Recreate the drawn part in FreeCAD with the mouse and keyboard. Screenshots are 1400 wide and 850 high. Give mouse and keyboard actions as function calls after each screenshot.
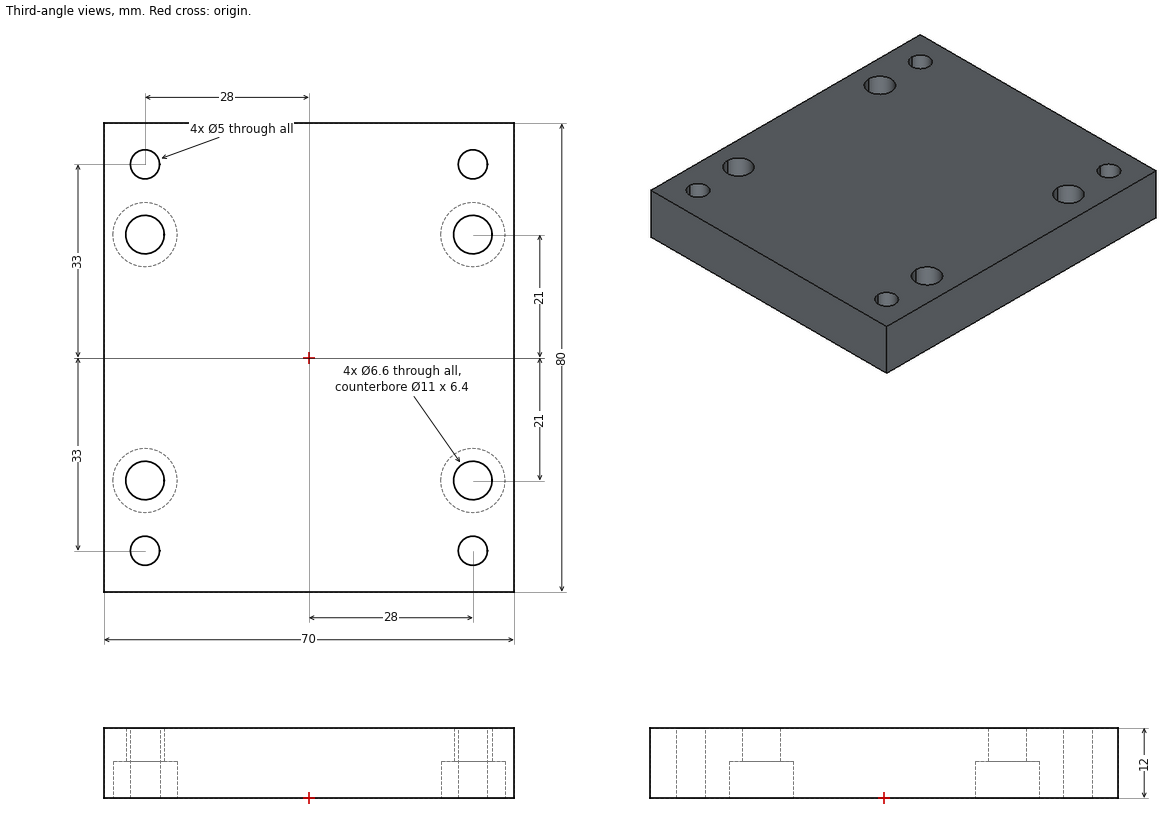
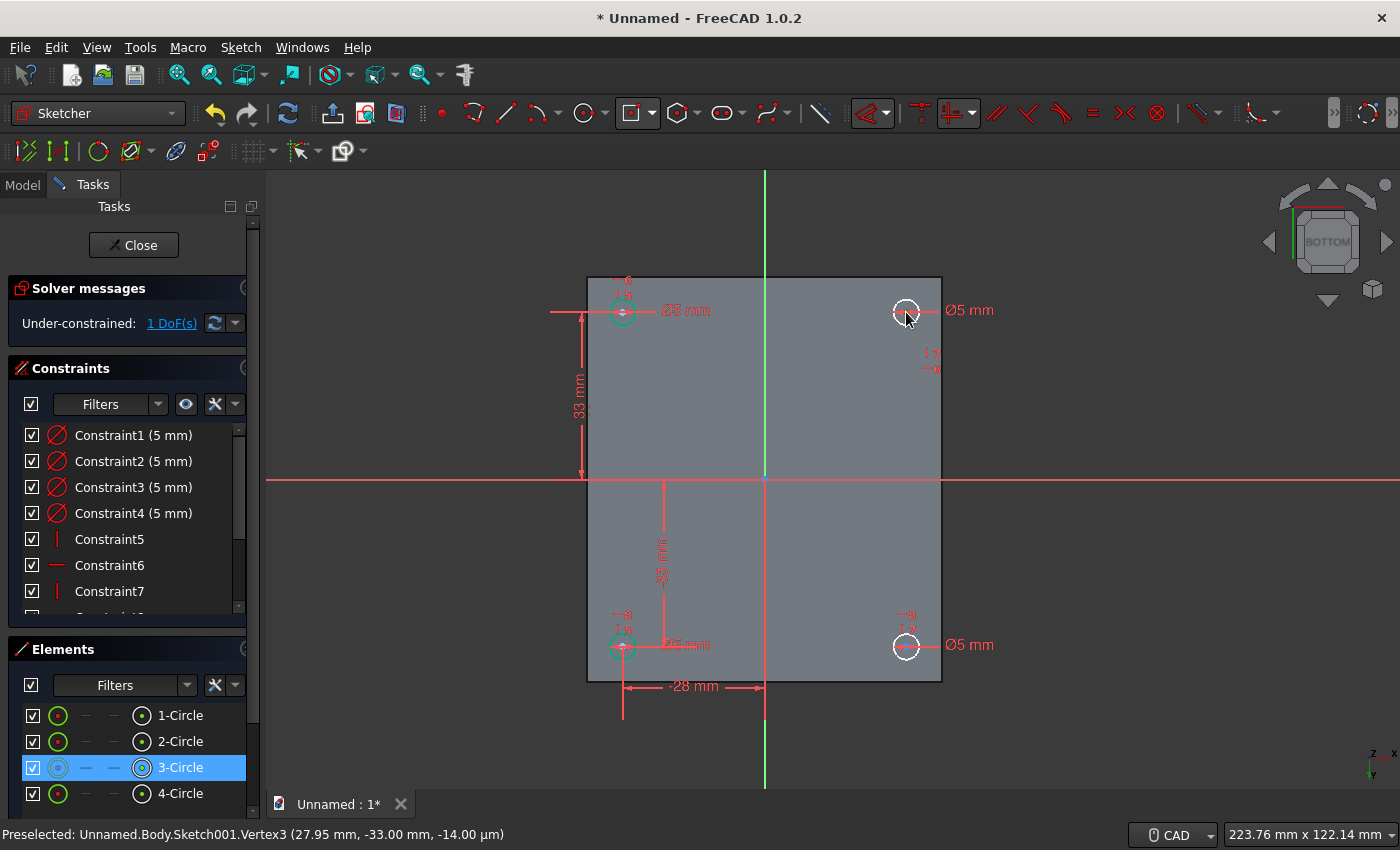
key(l)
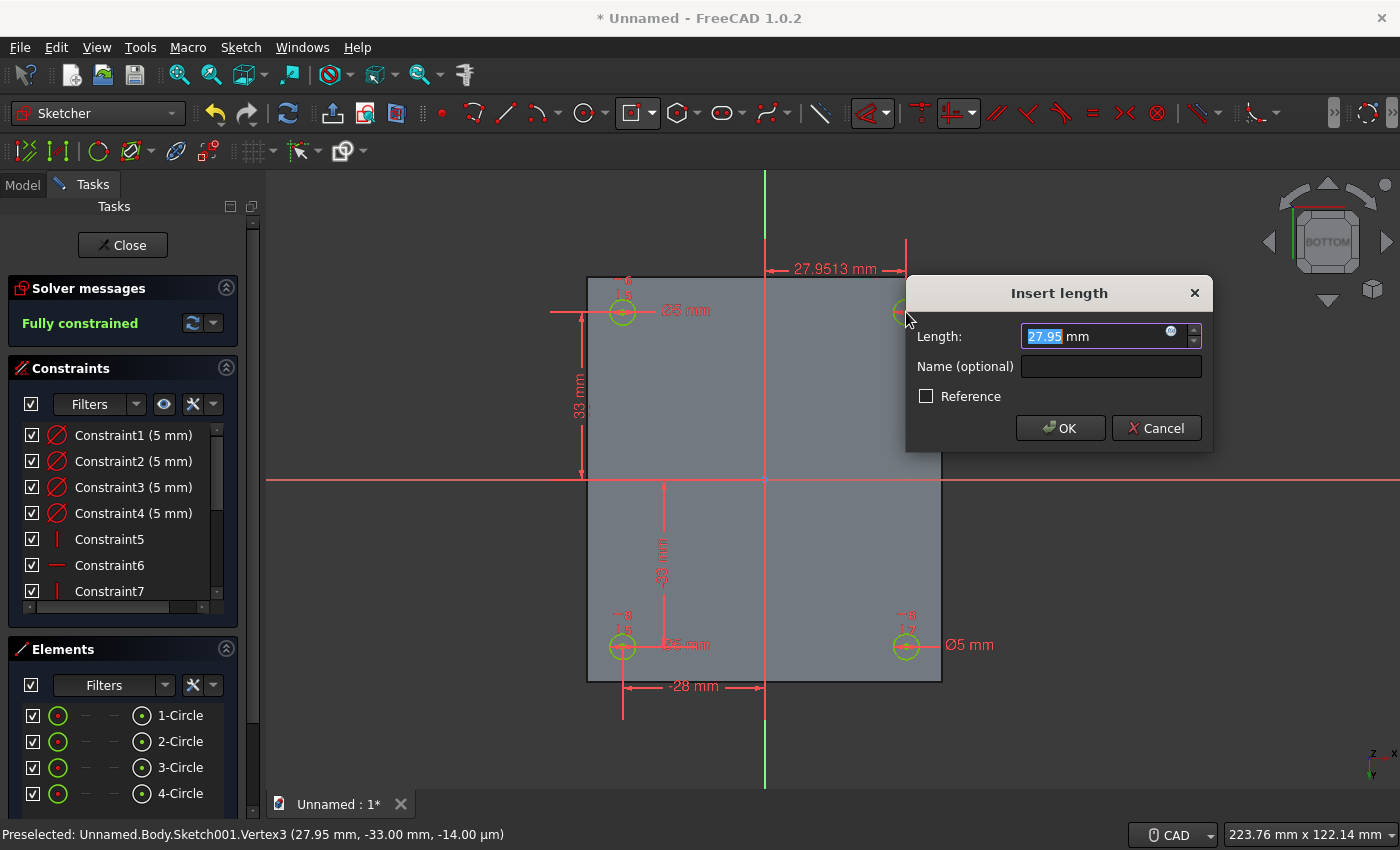
text(28)
key(Return)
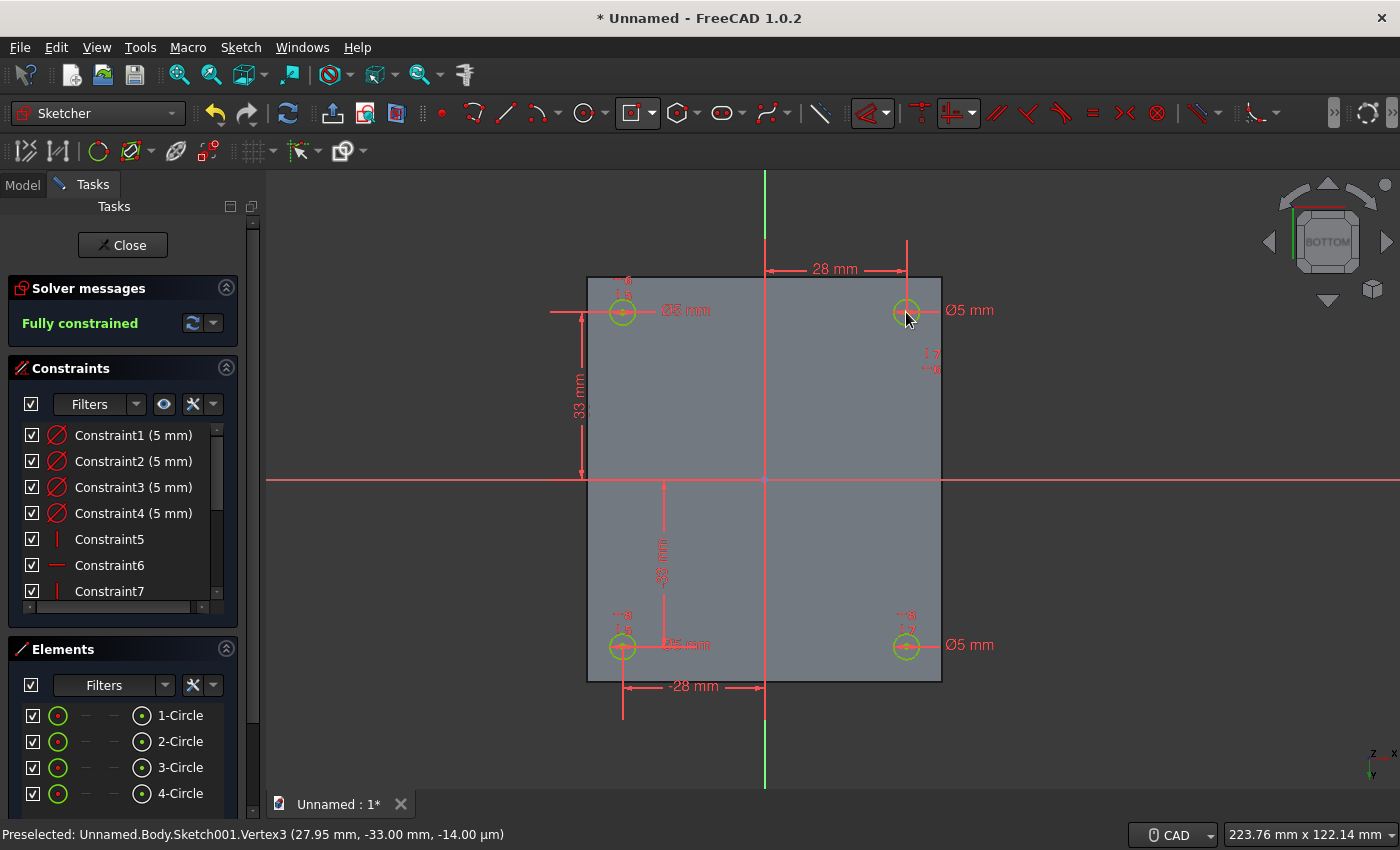
click(123, 245)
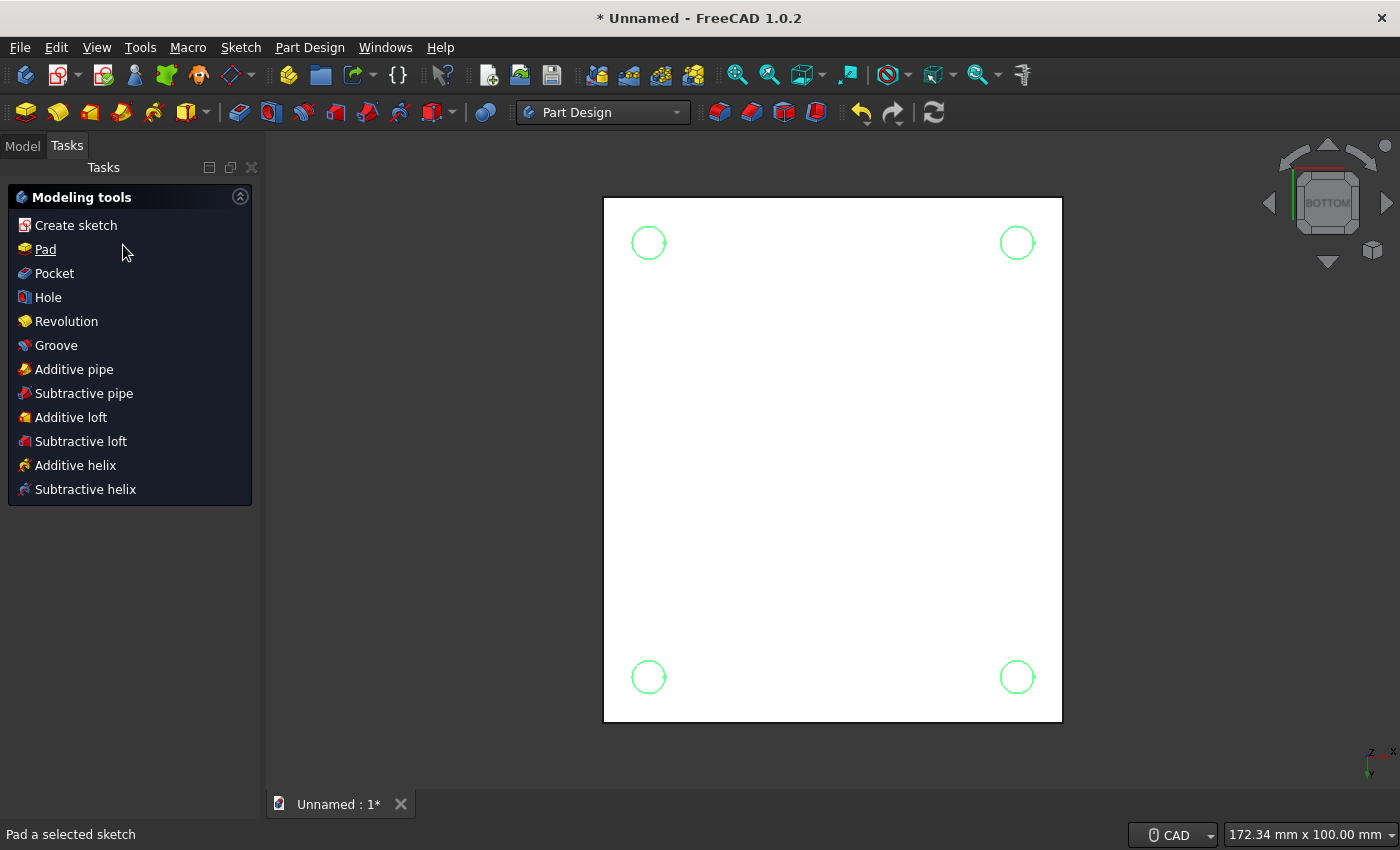
click(272, 112)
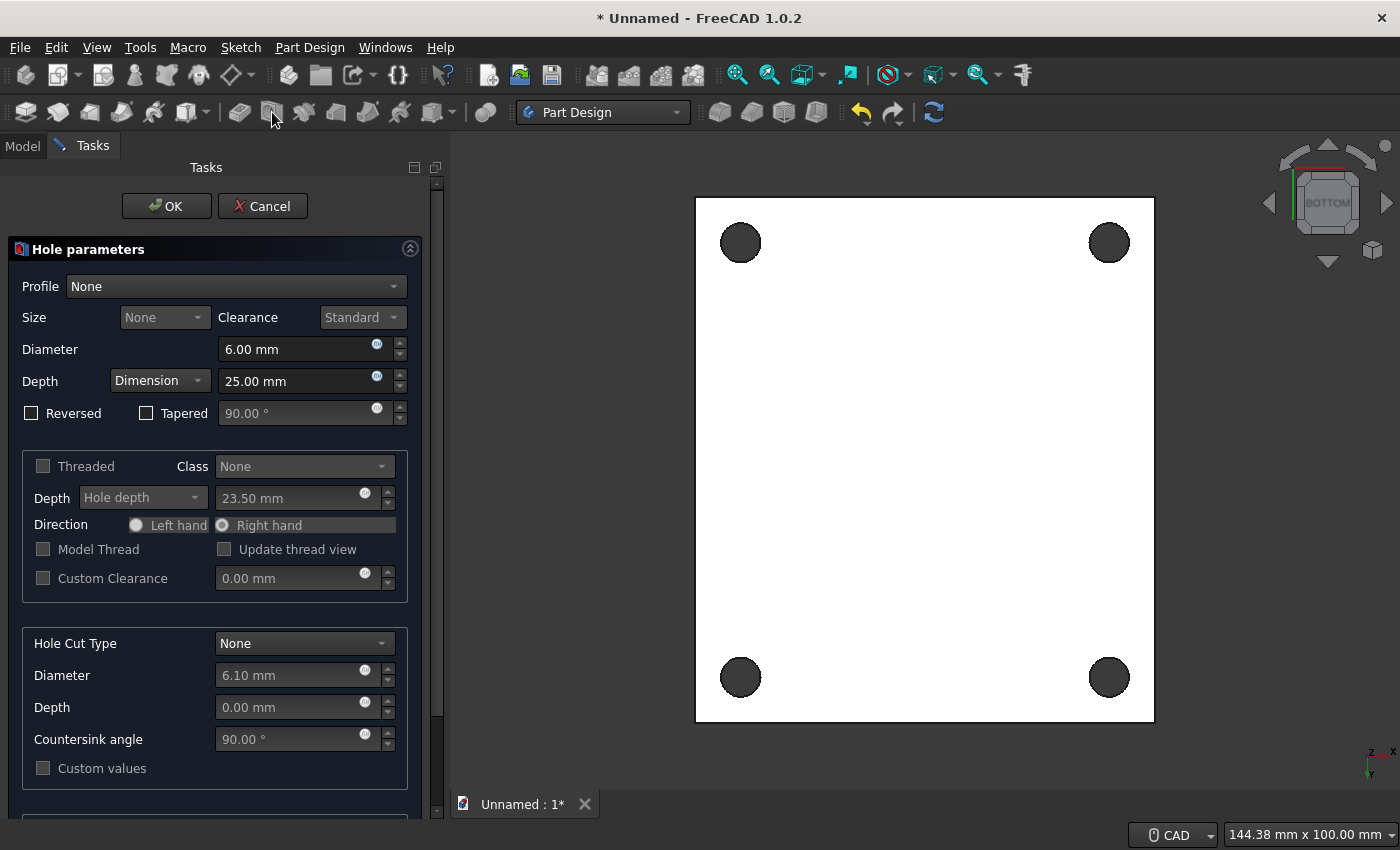
triple_click(305, 349)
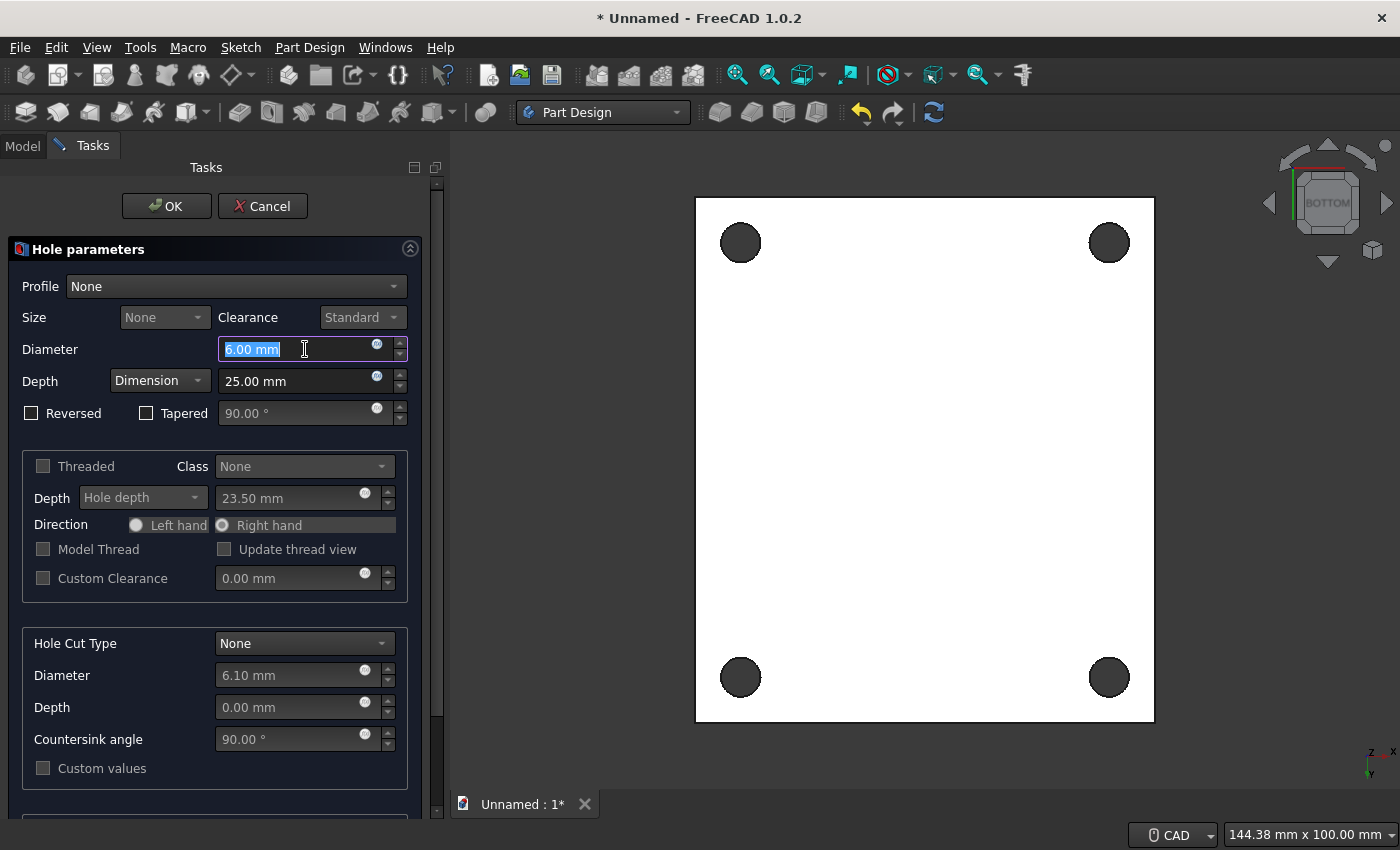
text(5)
key(Tab)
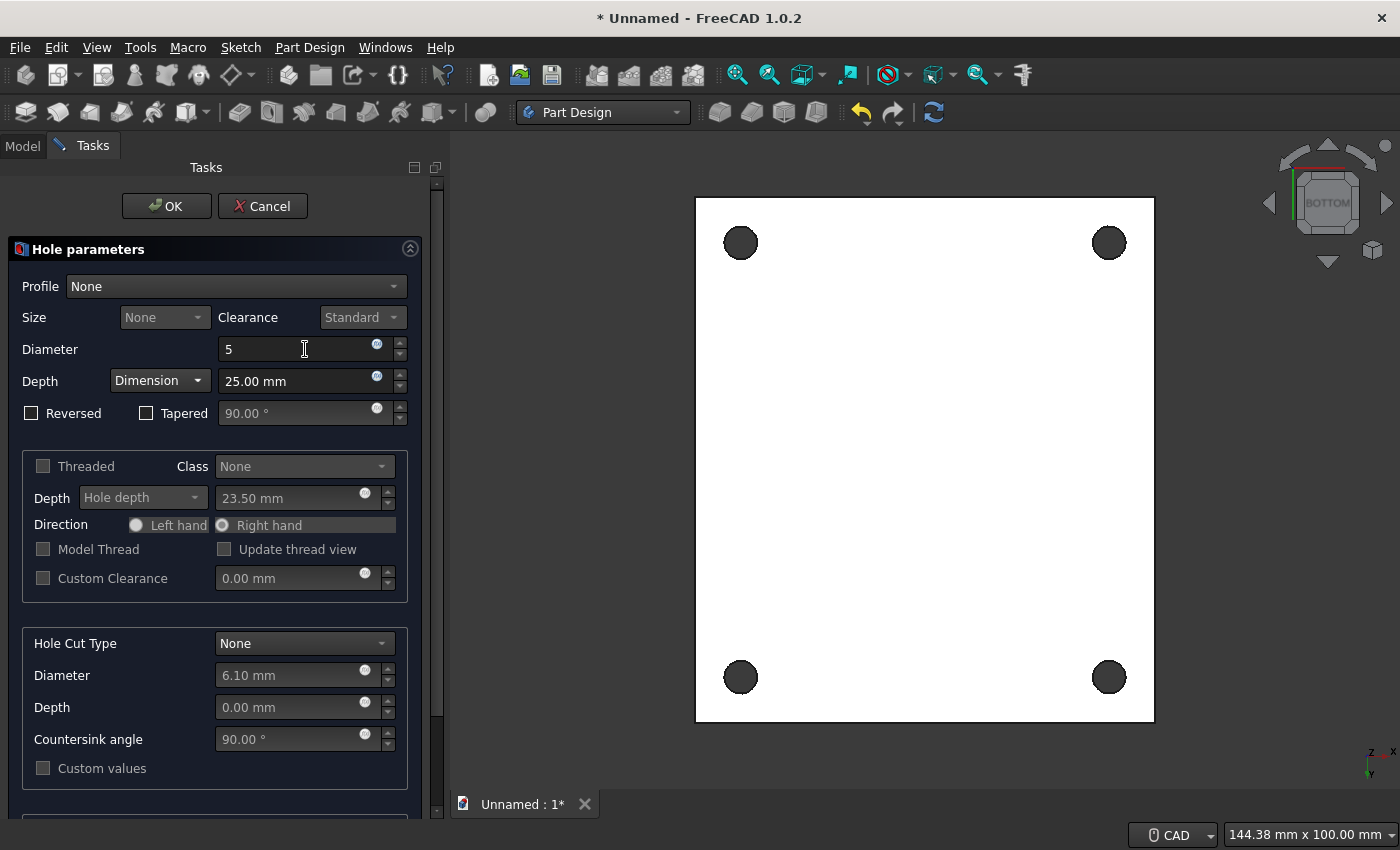
click(161, 380)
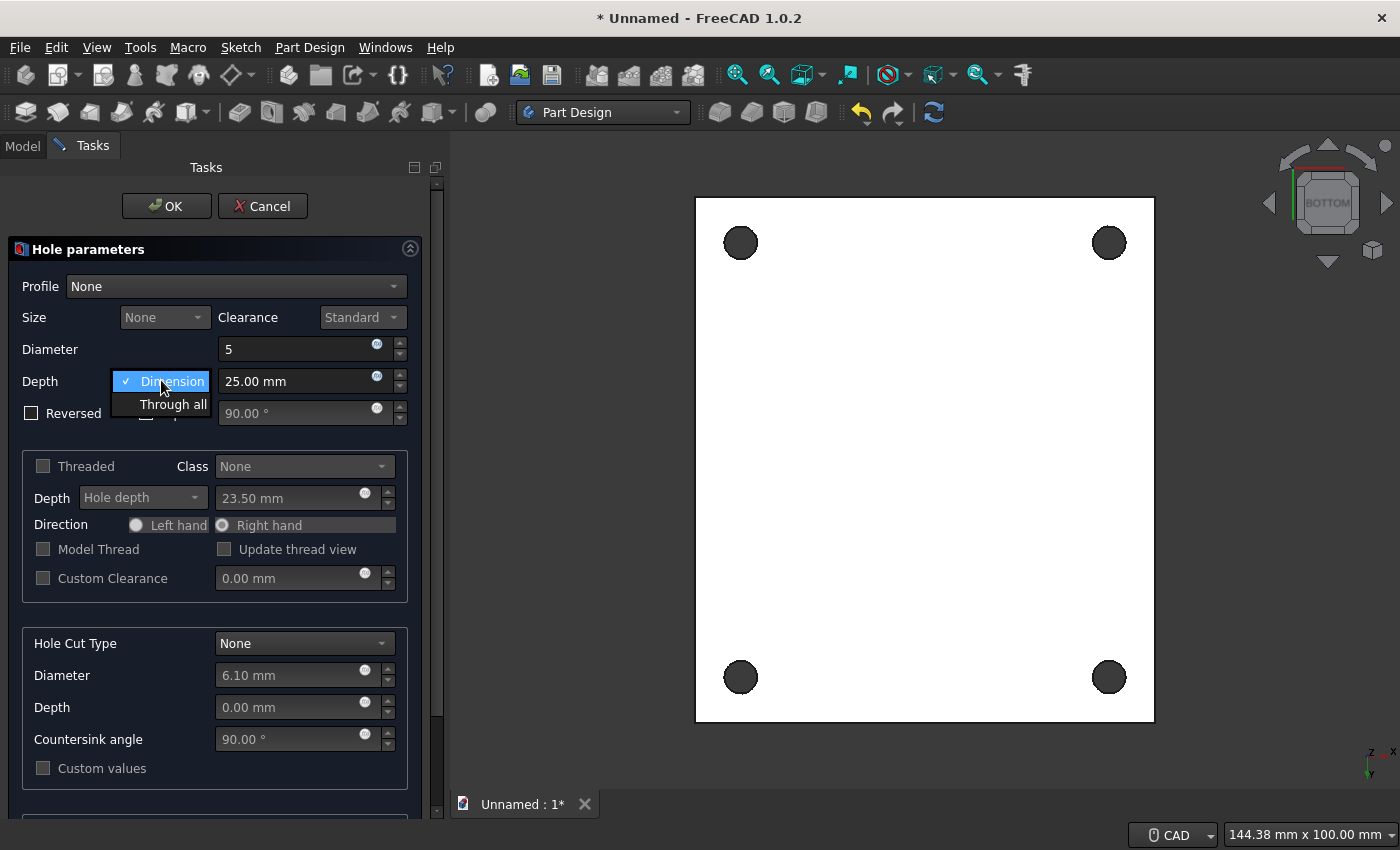
click(160, 404)